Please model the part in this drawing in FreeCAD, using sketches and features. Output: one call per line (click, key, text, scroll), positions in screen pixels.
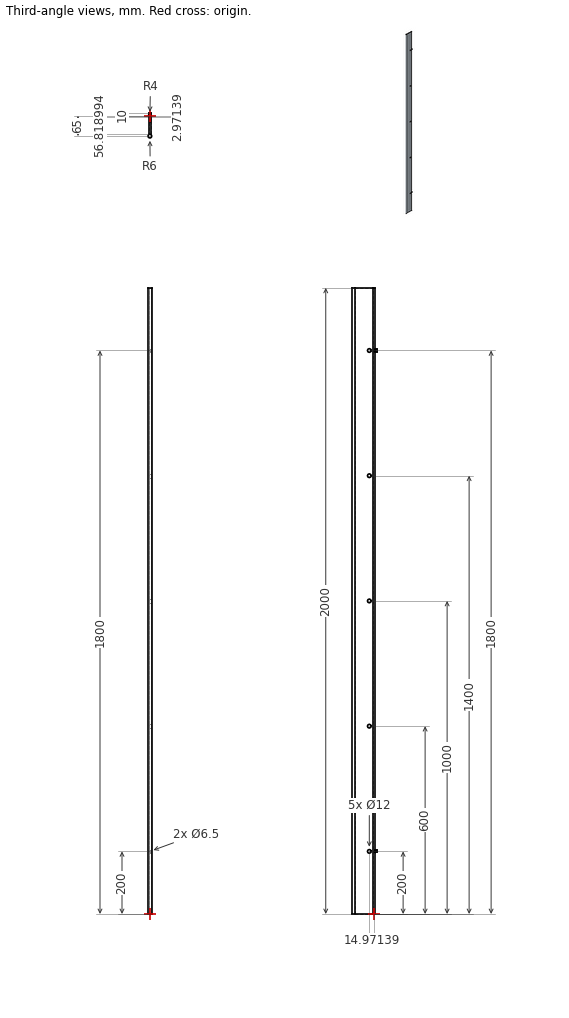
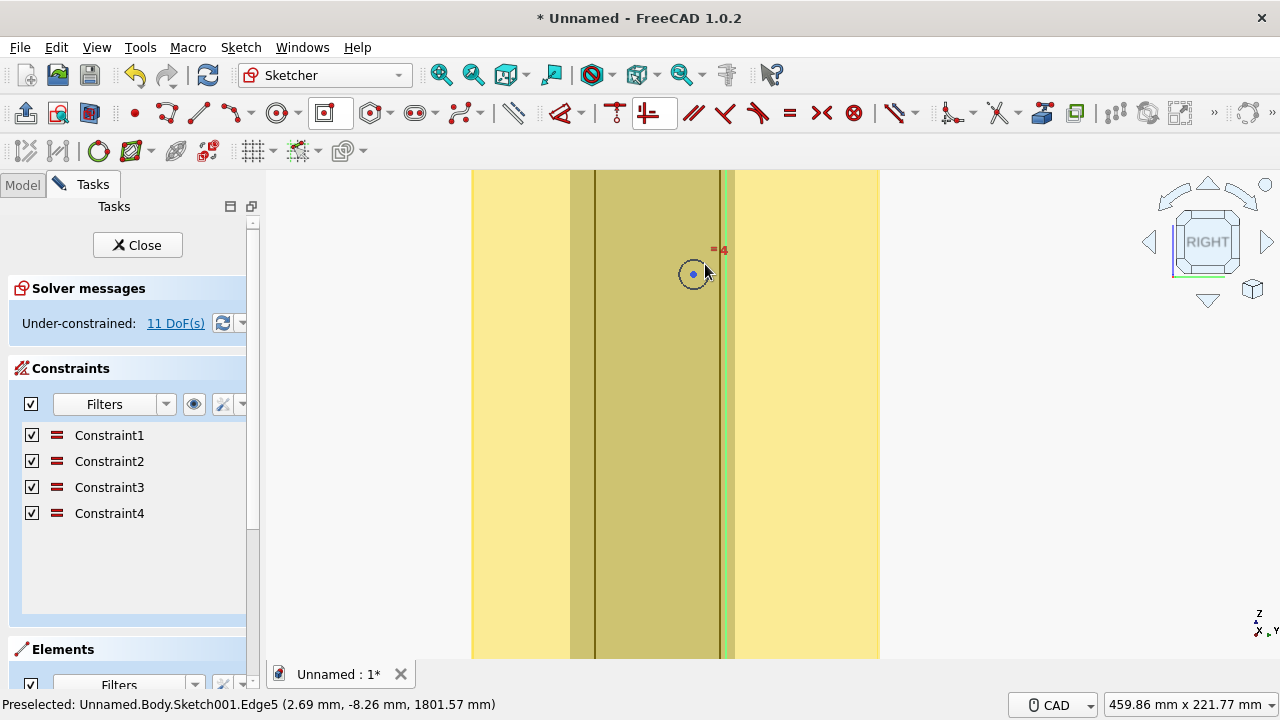
scroll(705, 267, down, 13)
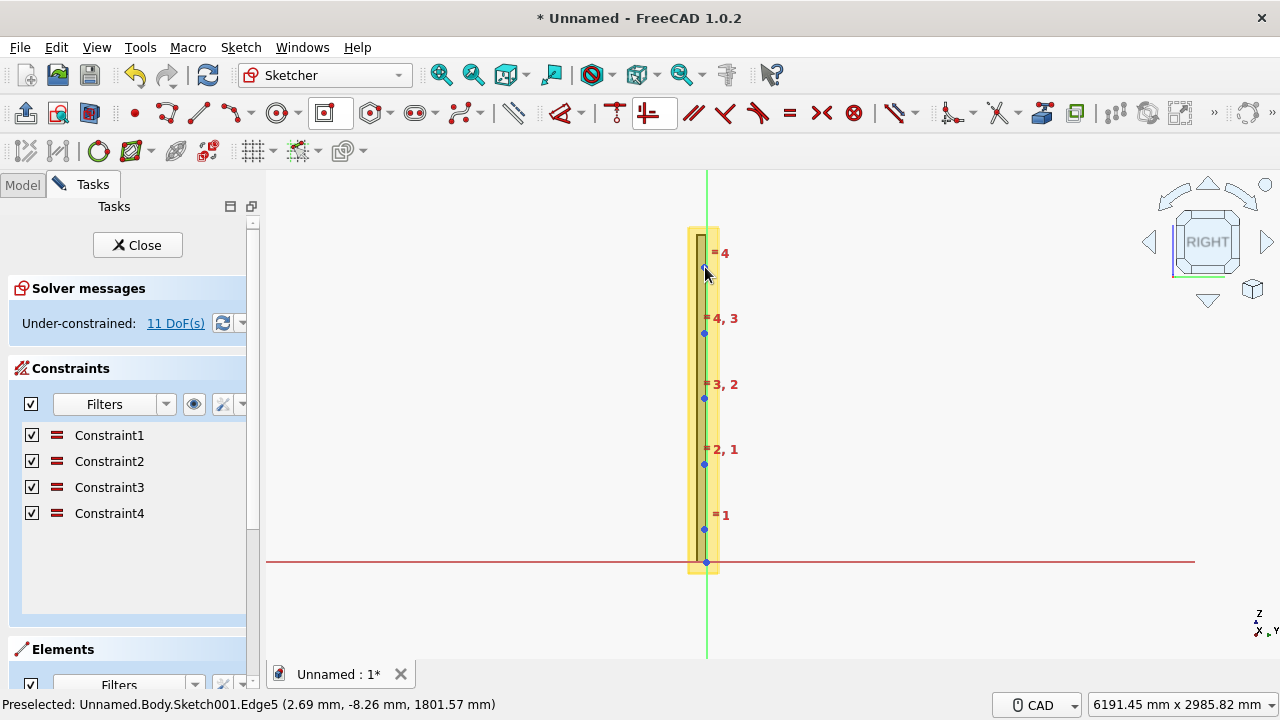
click(705, 530)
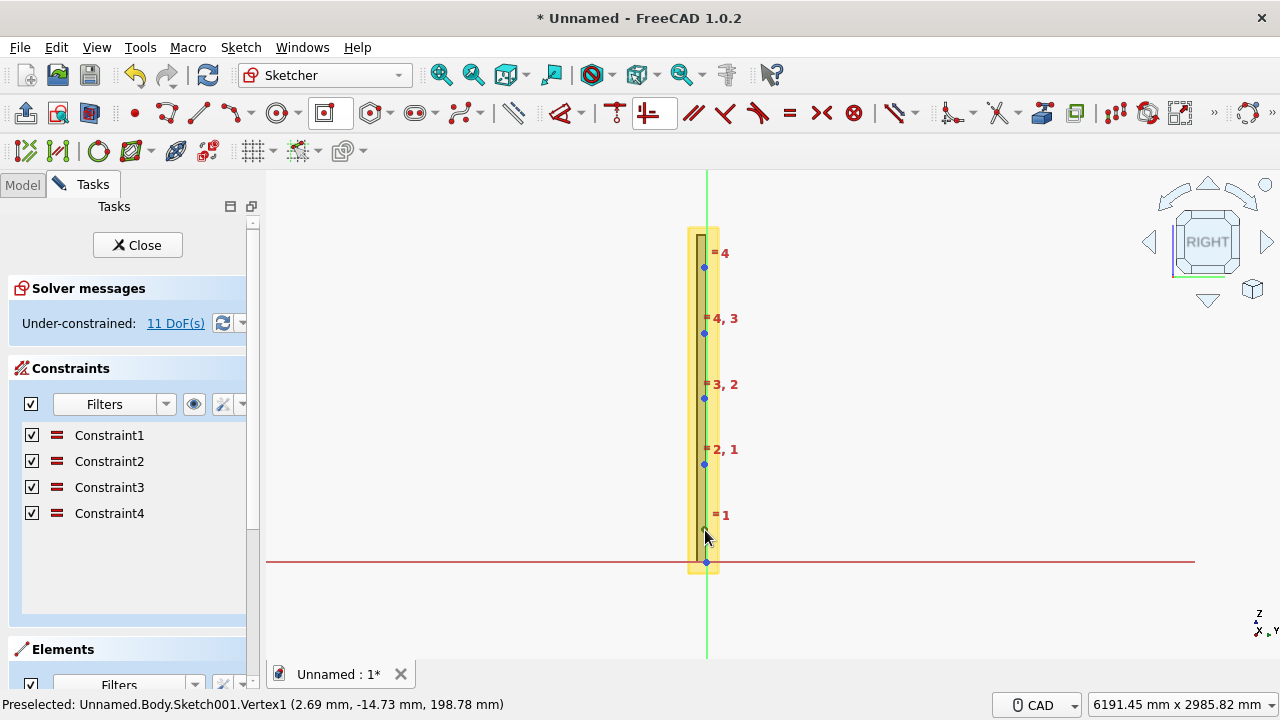
click(705, 464)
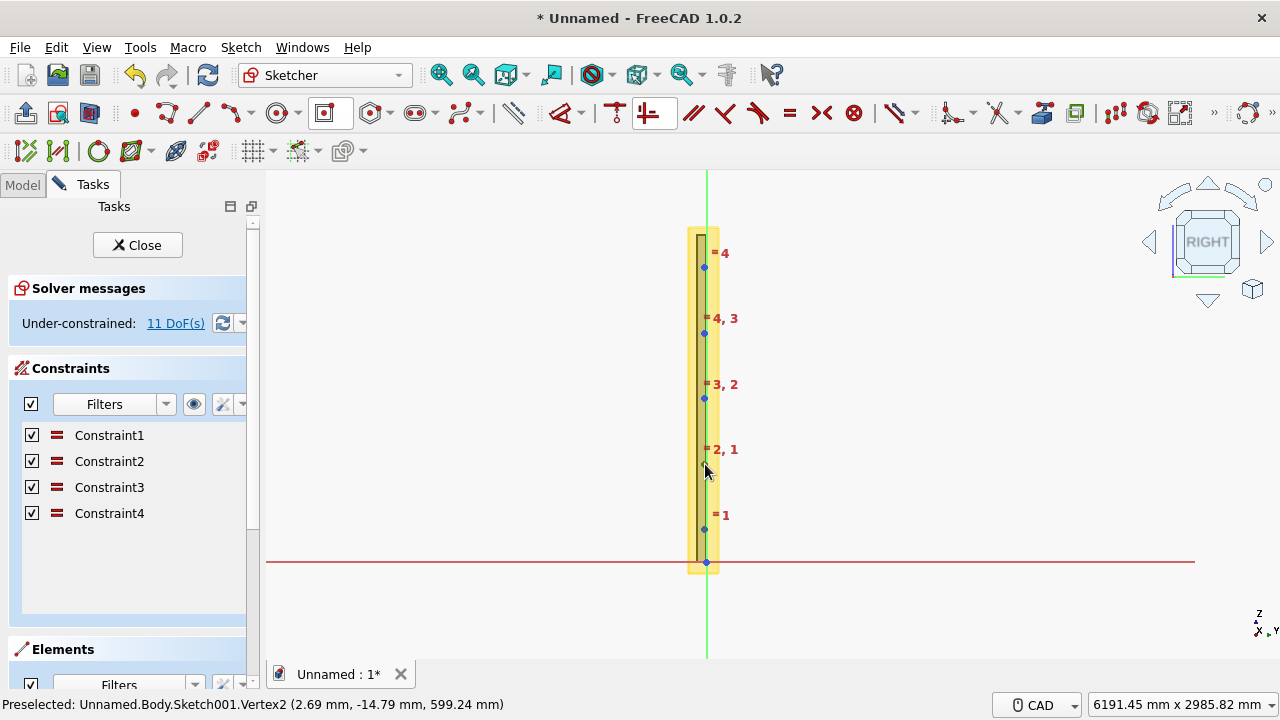
key(v)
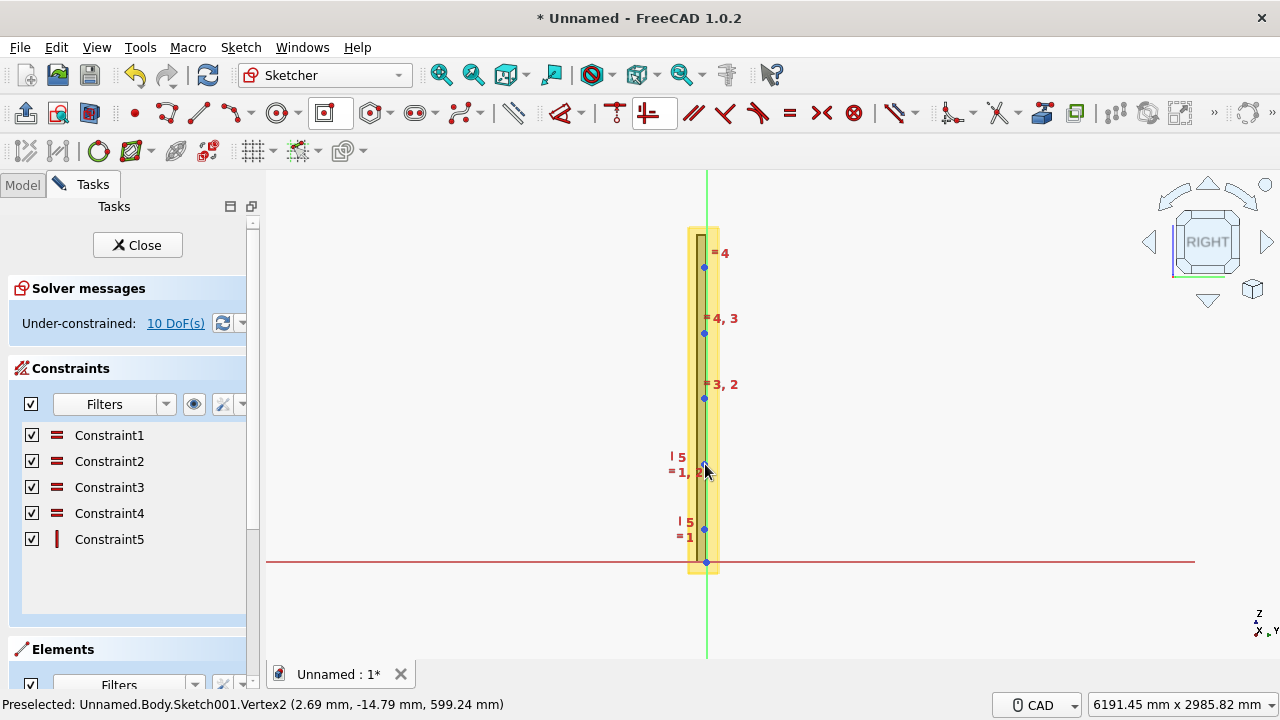
click(705, 464)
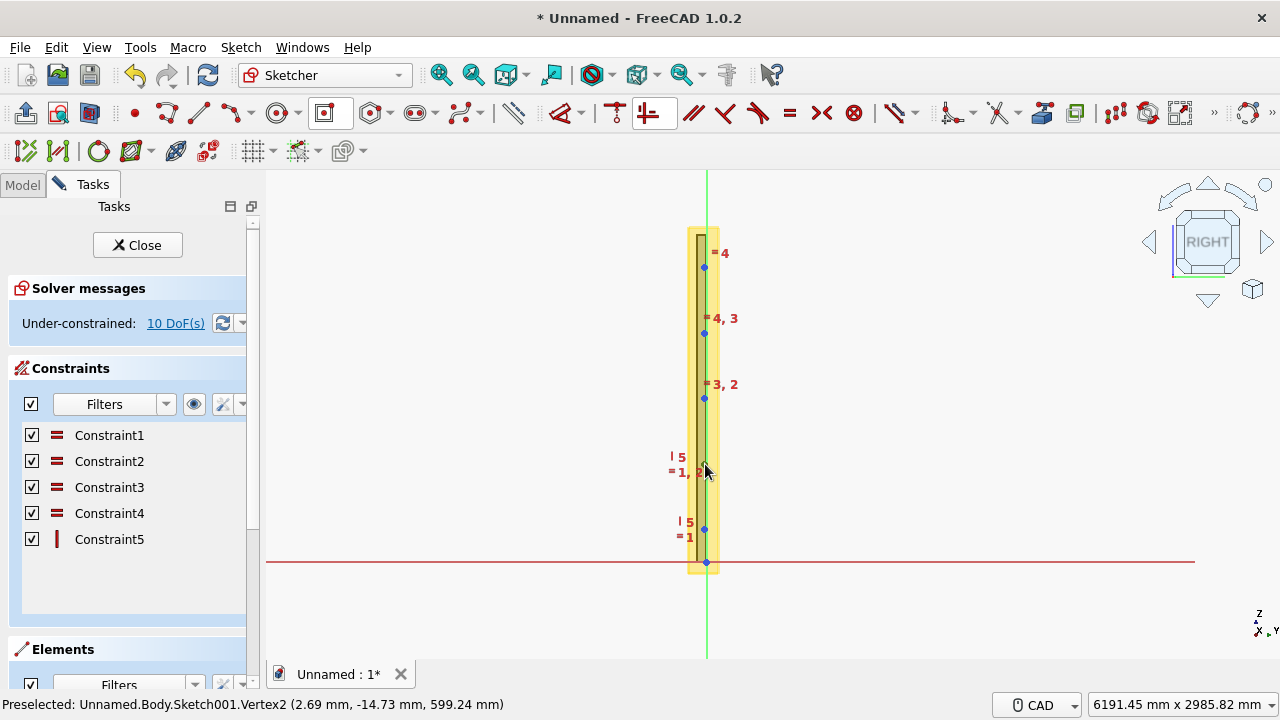
click(705, 399)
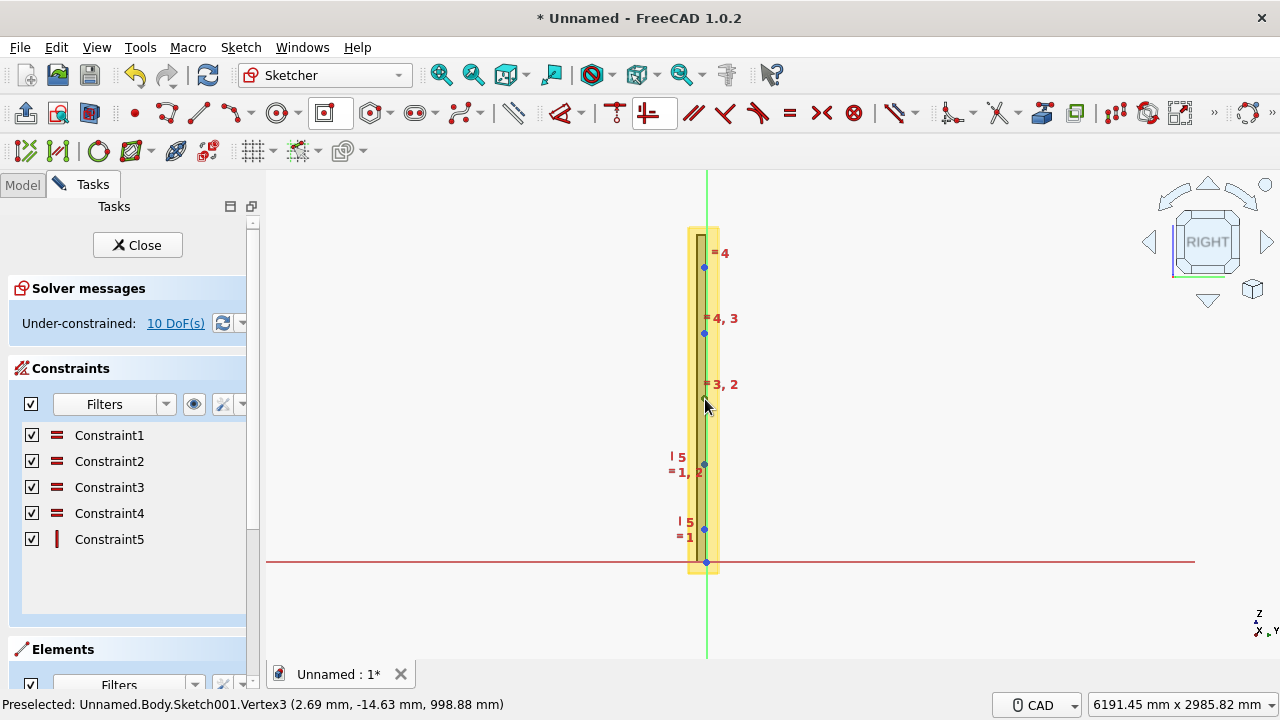
key(v)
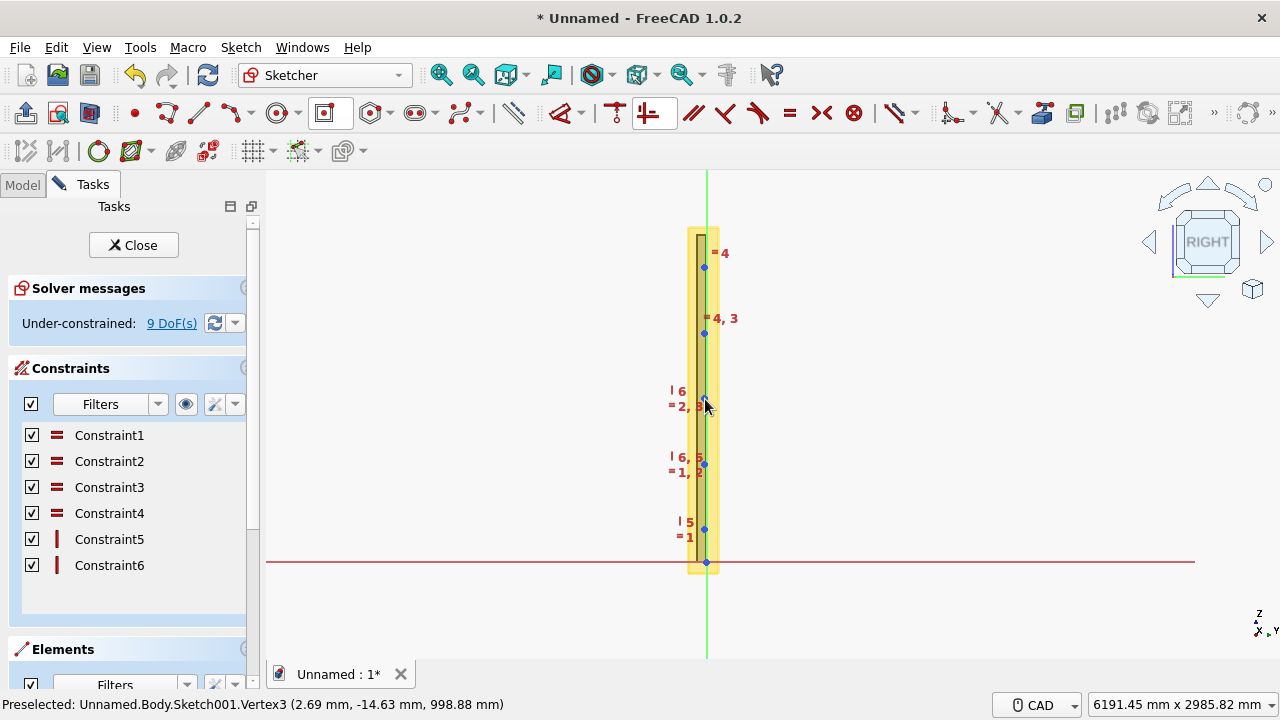
click(705, 399)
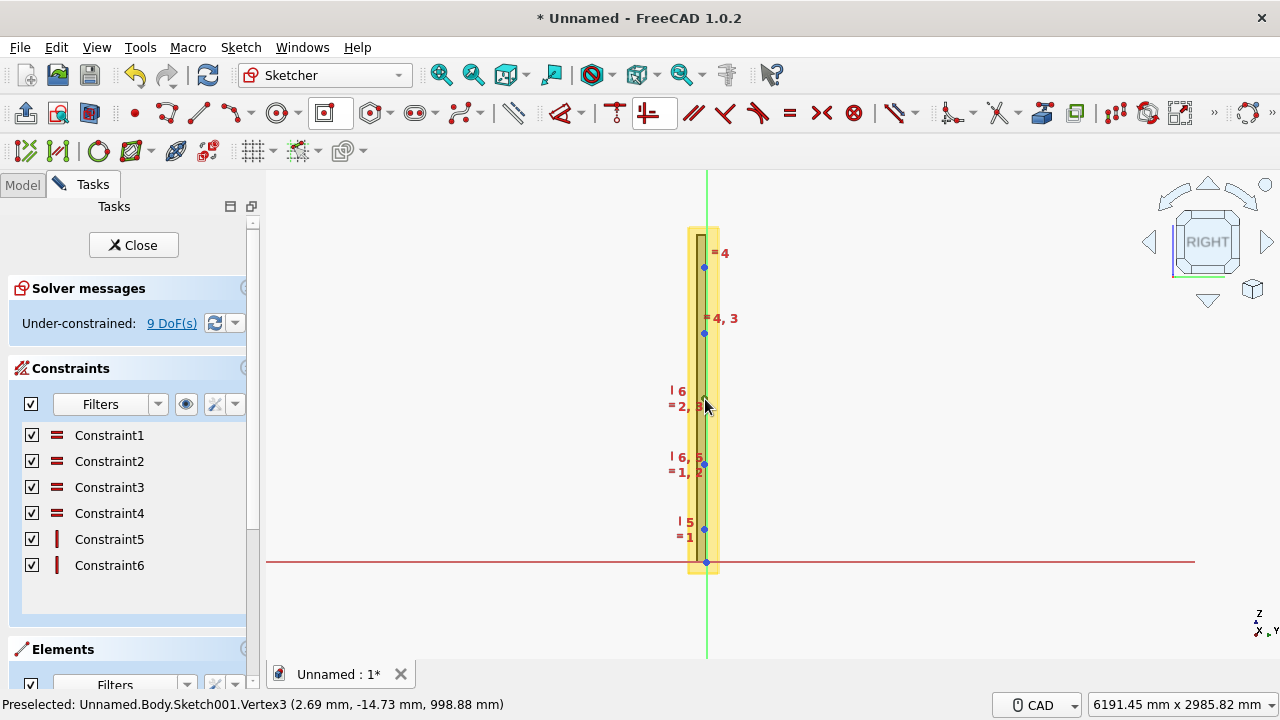
click(705, 333)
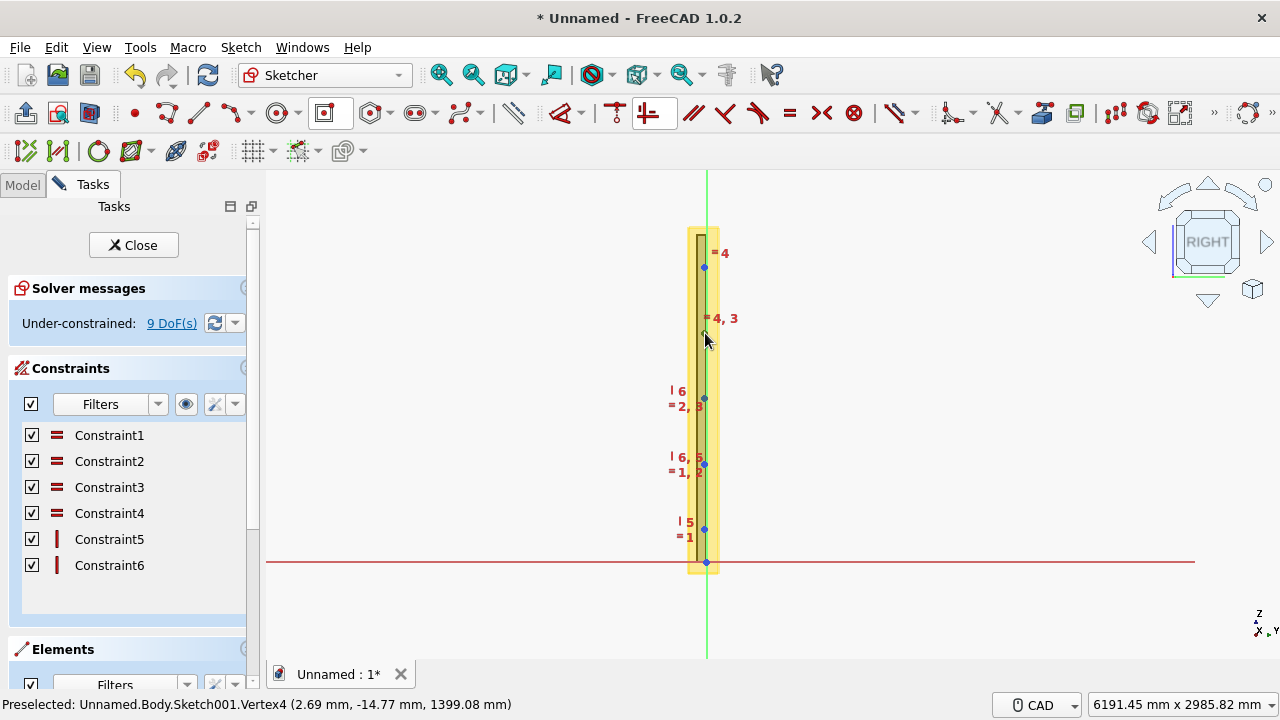
click(672, 114)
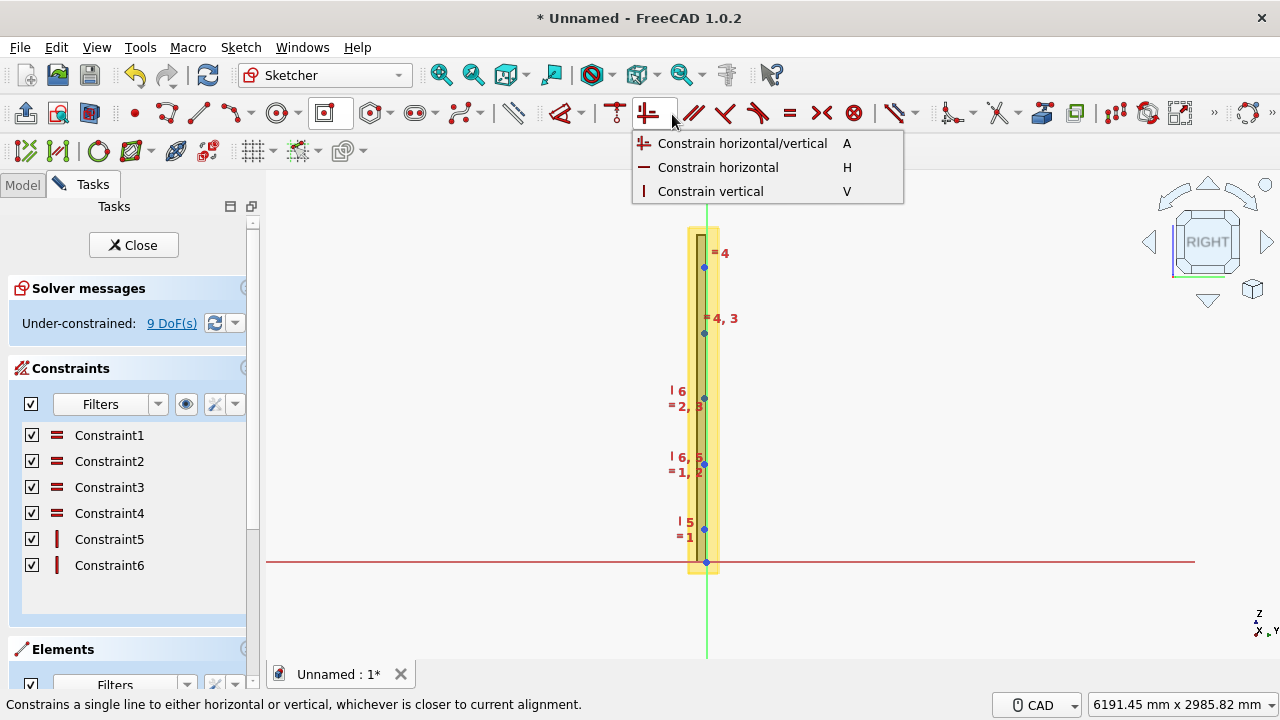
click(768, 191)